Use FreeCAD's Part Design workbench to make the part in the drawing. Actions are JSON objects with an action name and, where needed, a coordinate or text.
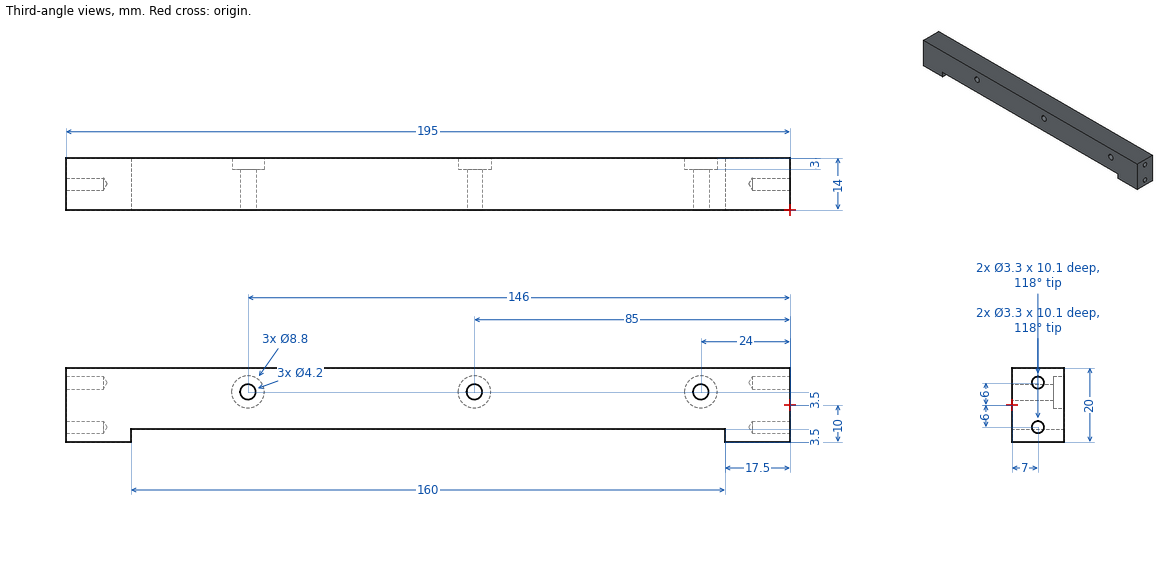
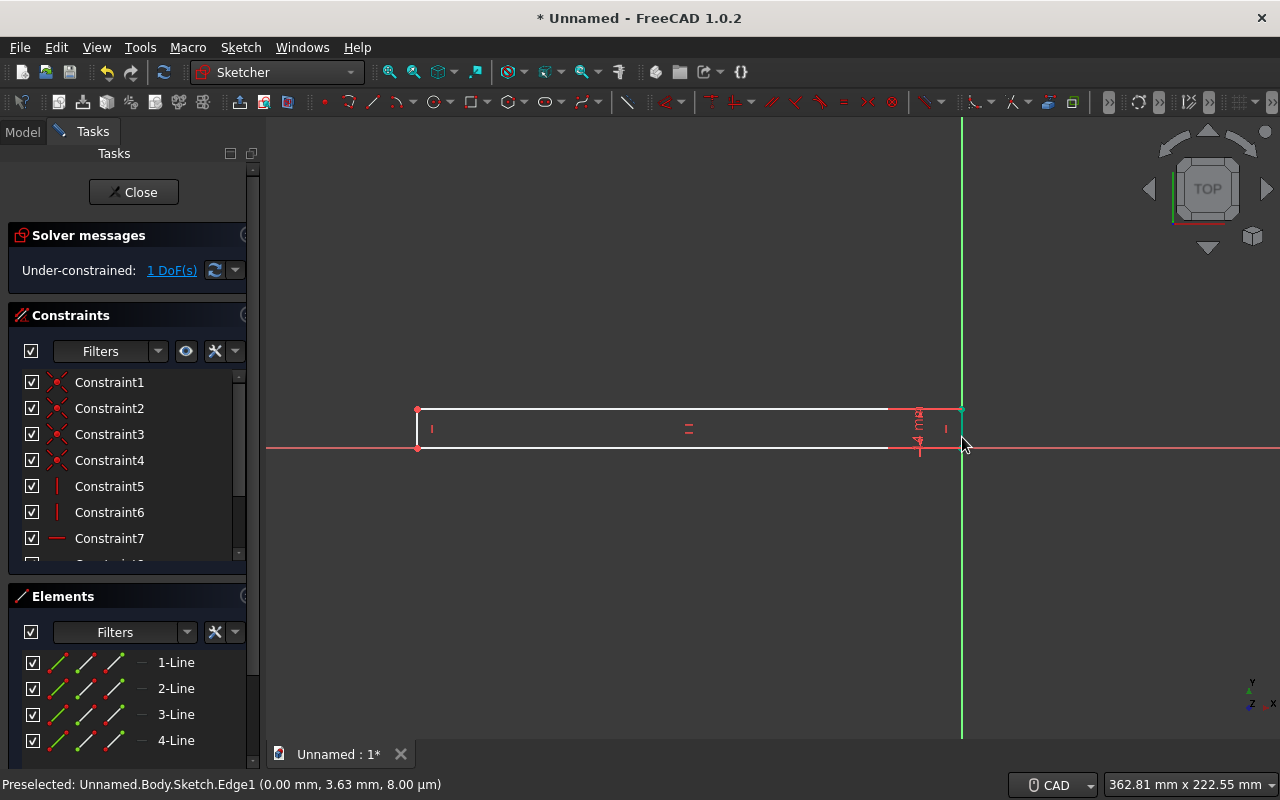
{"action": "left_click", "coordinate": [798, 409]}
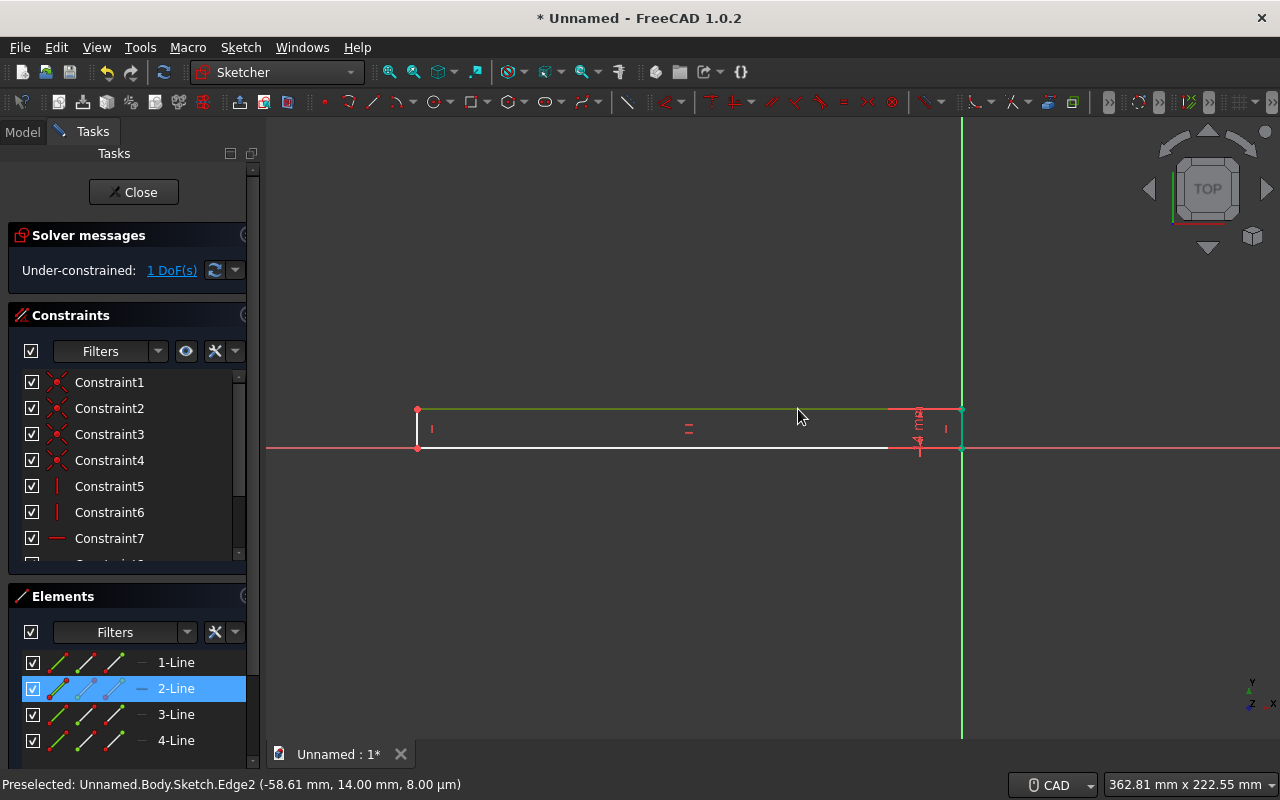
{"action": "key", "text": "l"}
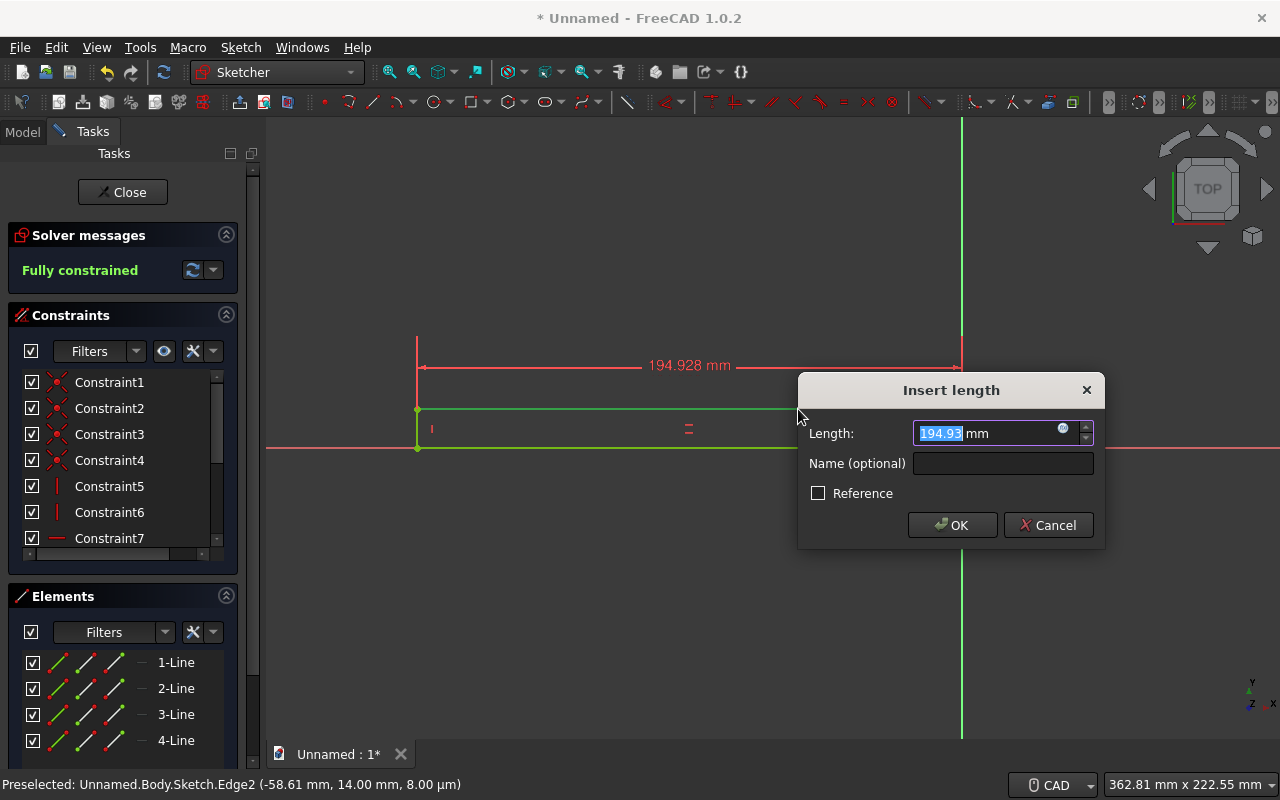
{"action": "type", "text": "195"}
{"action": "key", "text": "Return"}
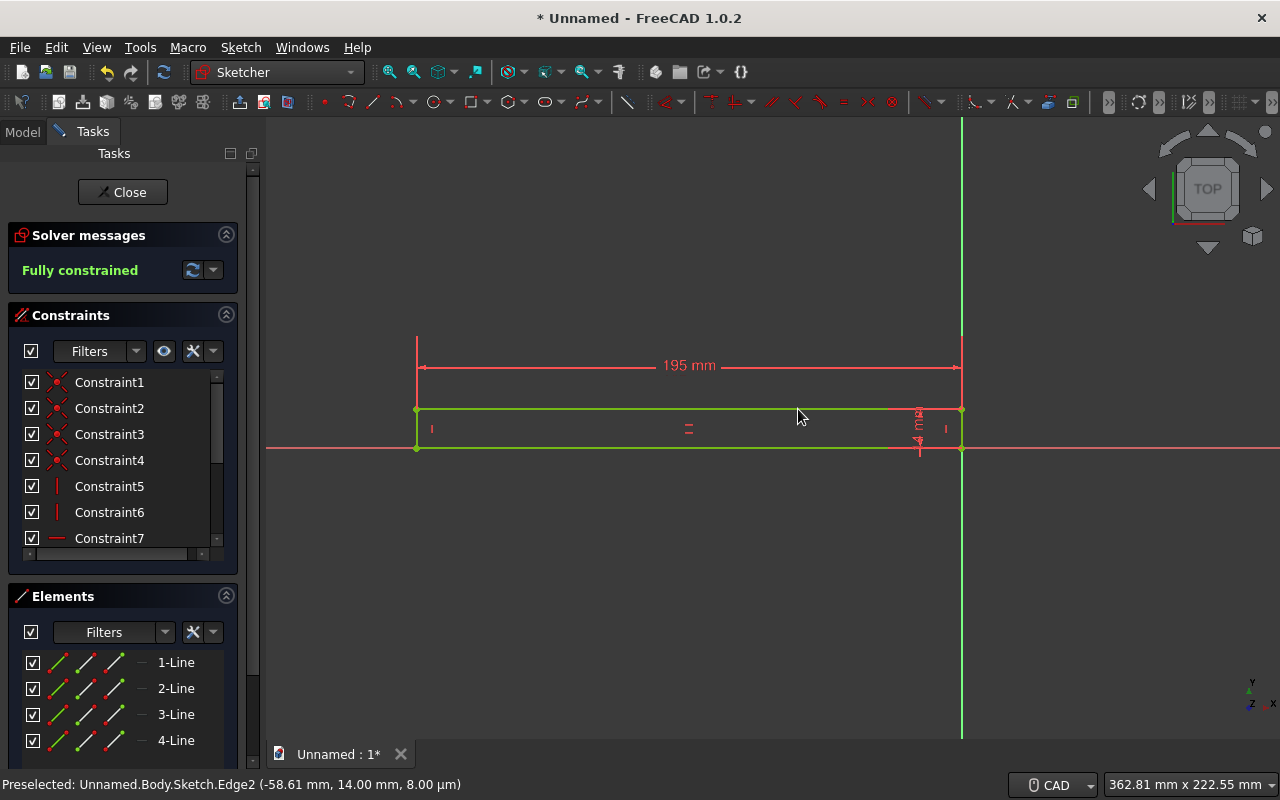
{"action": "left_click", "coordinate": [123, 192]}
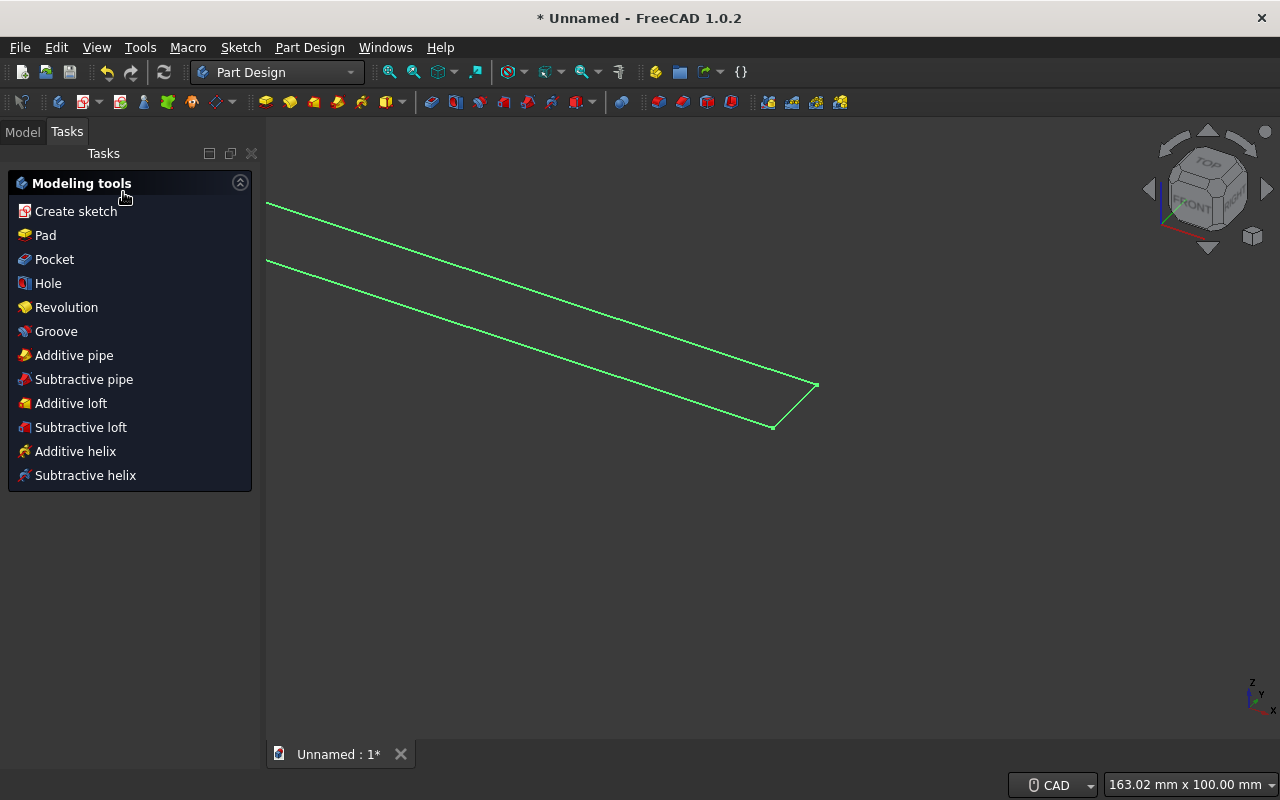
{"action": "left_click", "coordinate": [266, 102]}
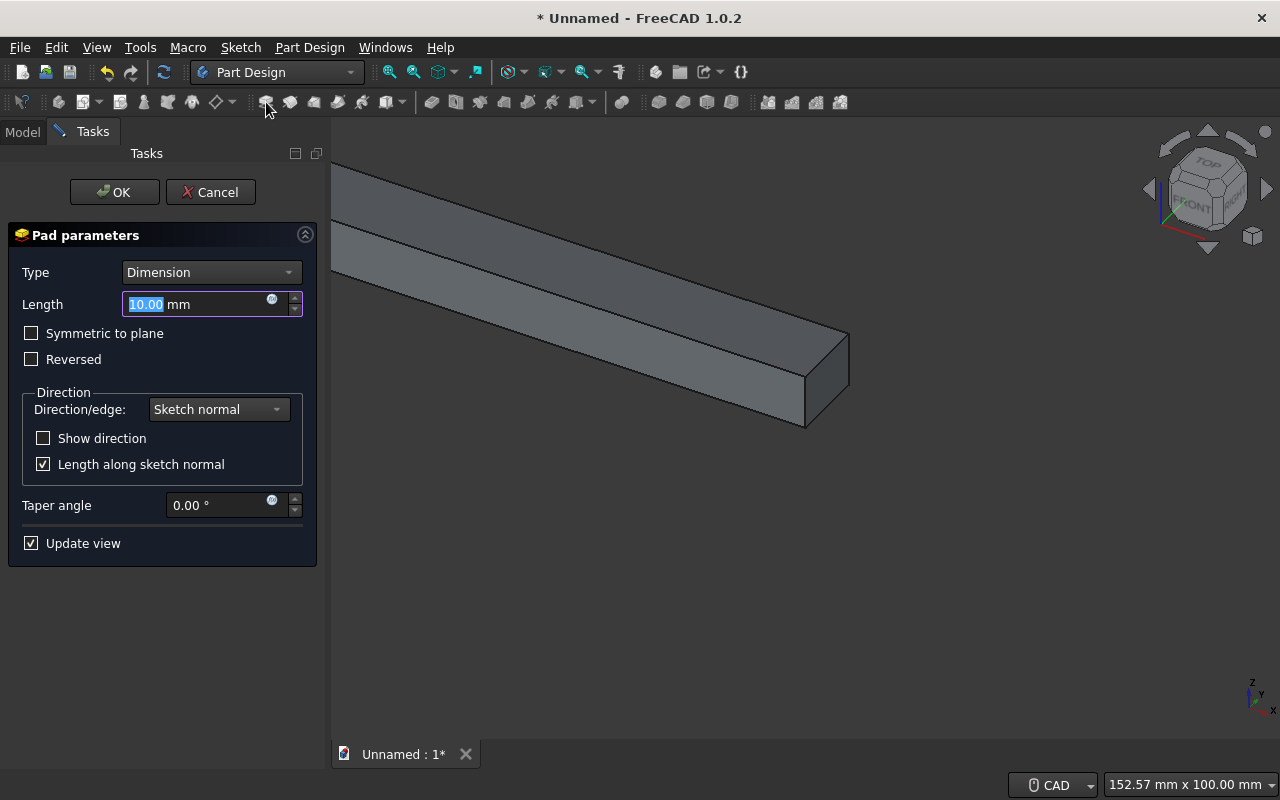
{"action": "type", "text": "20"}
{"action": "key", "text": "Tab"}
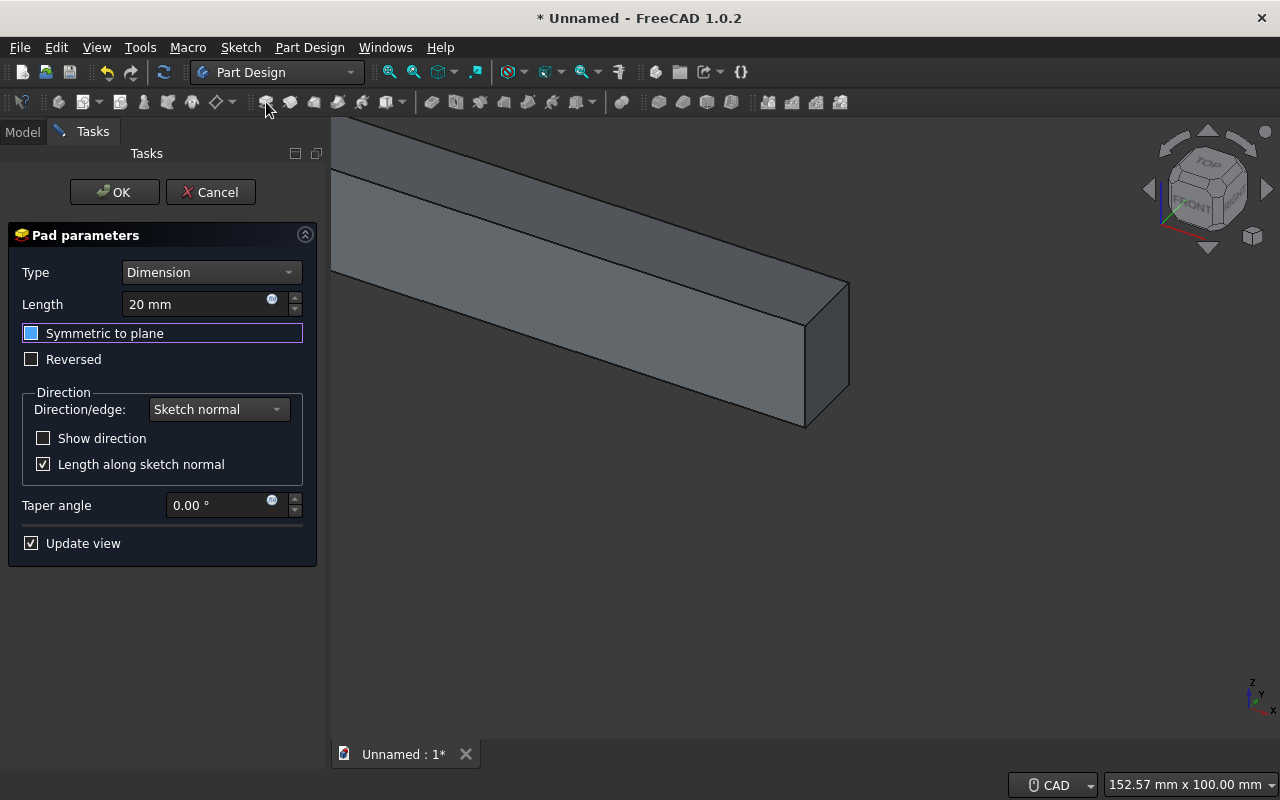
{"action": "left_click", "coordinate": [30, 333]}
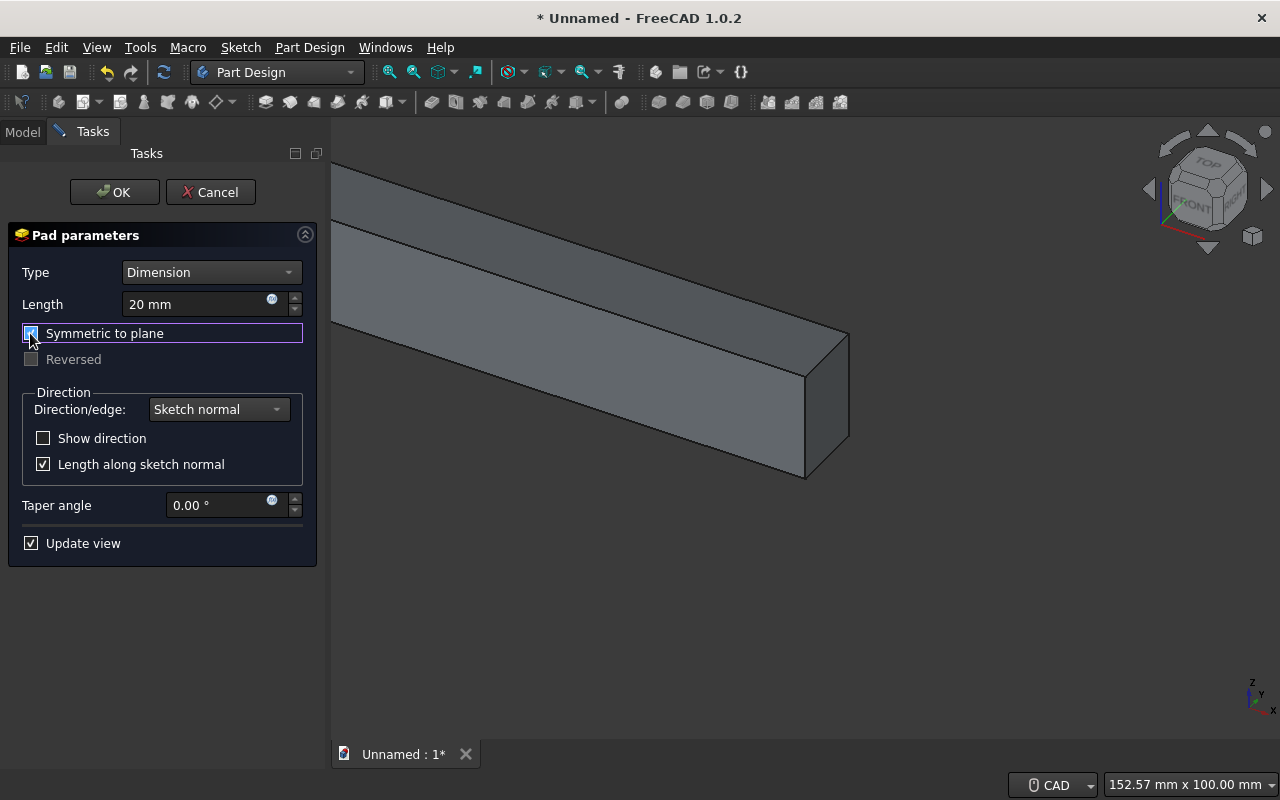
{"action": "left_click", "coordinate": [115, 192]}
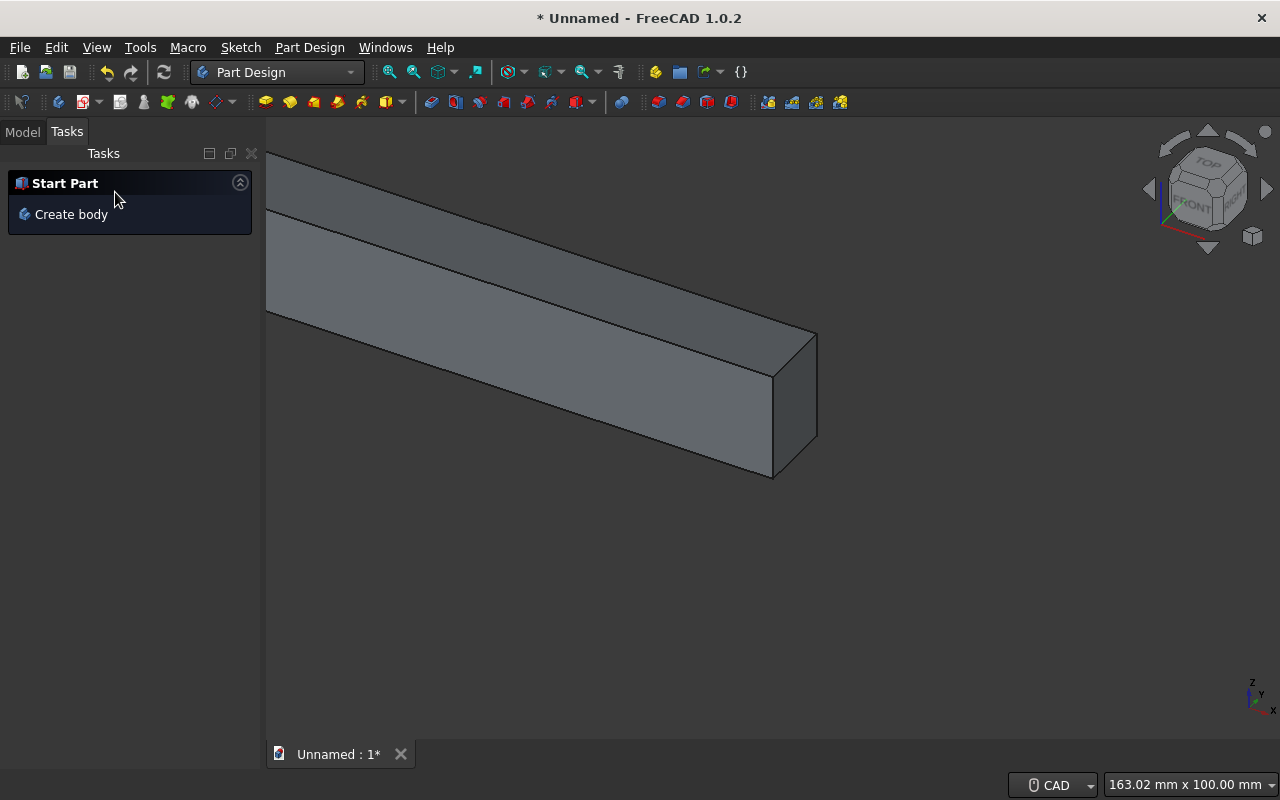
{"action": "key", "text": "v f"}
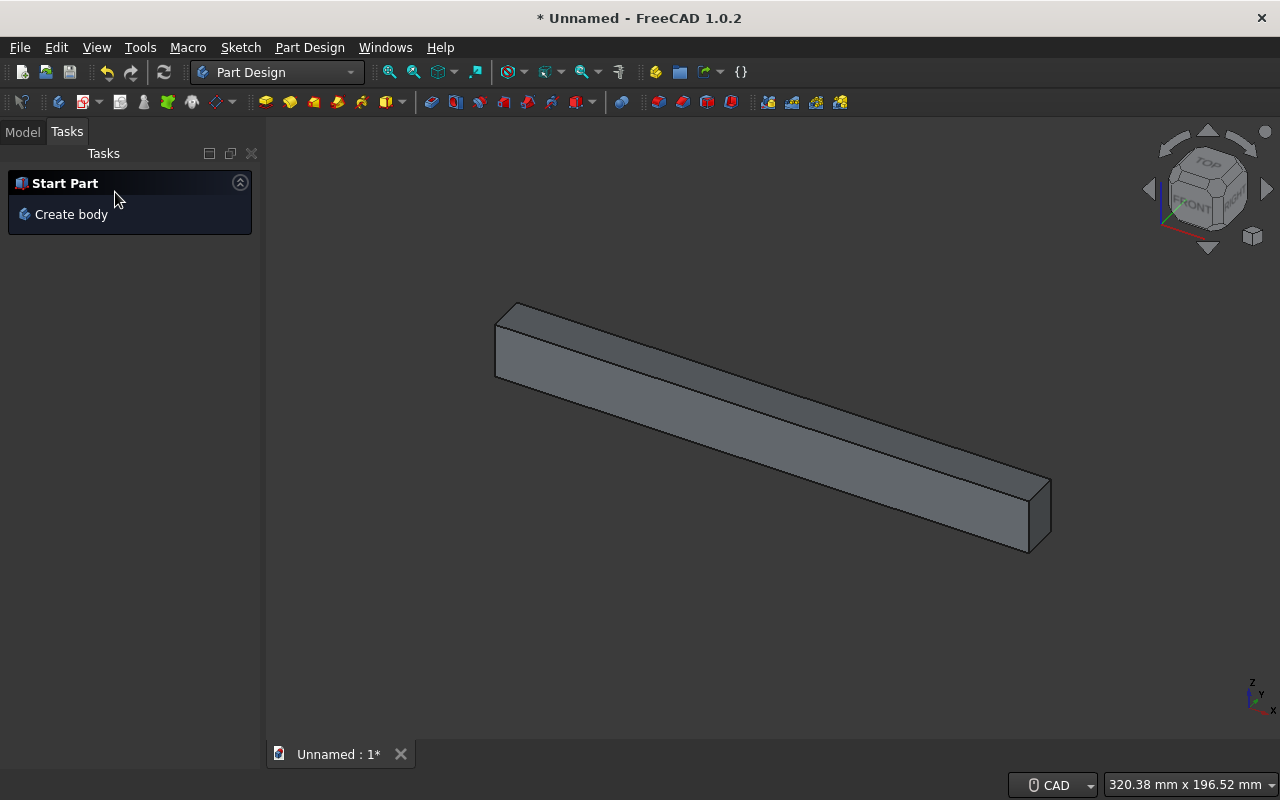
{"action": "key", "text": "6"}